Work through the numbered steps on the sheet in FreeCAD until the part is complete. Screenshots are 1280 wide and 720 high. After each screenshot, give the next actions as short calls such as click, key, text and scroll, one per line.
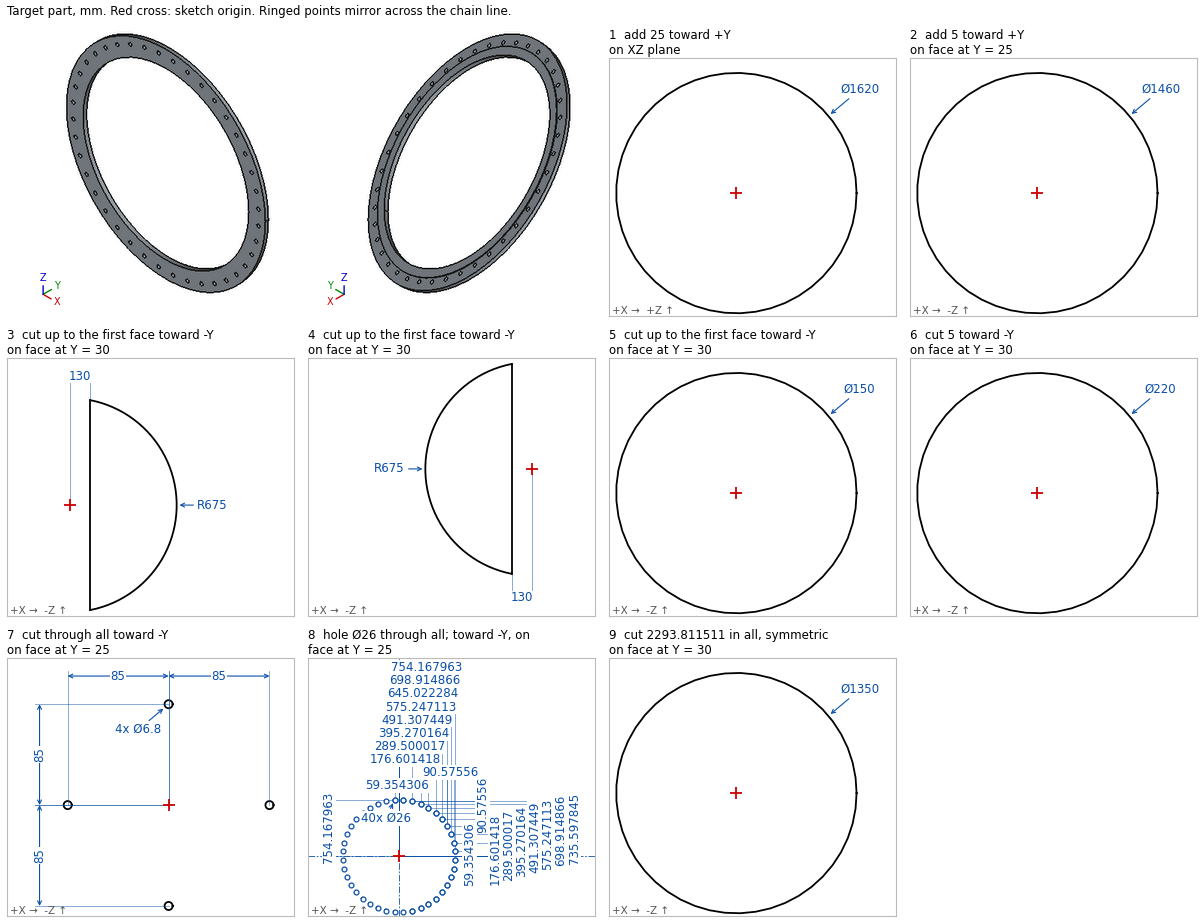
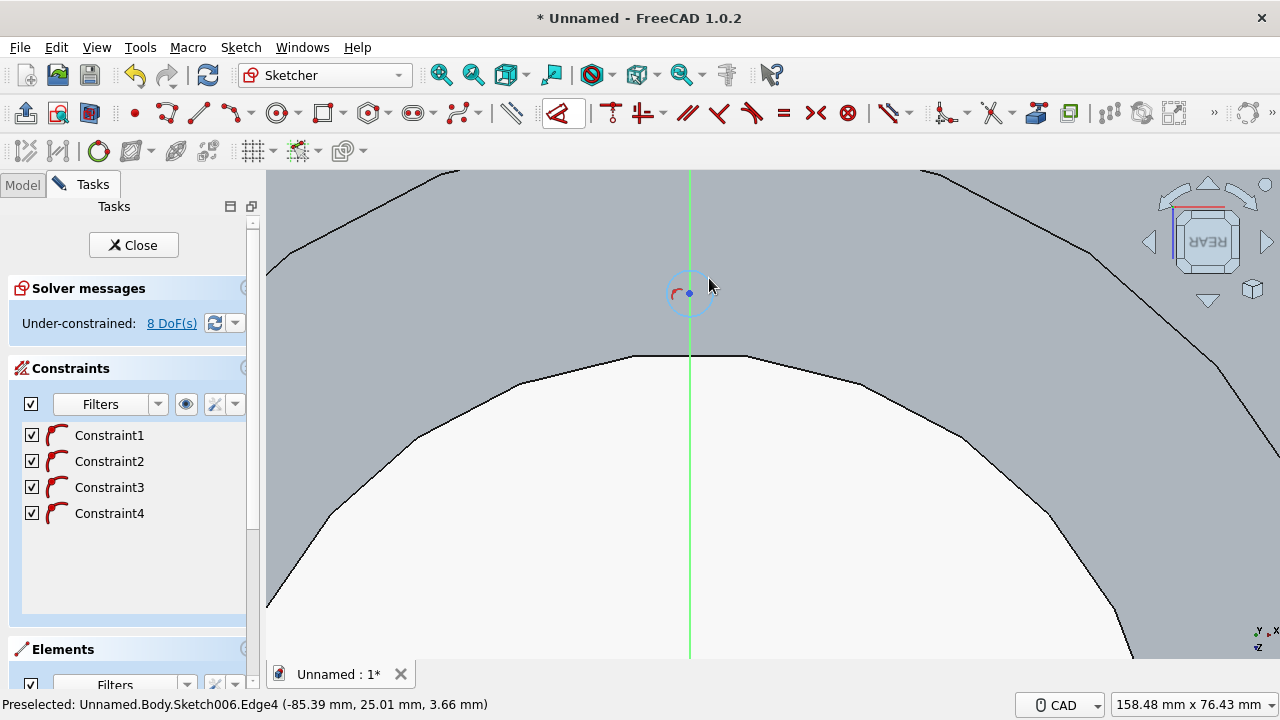
click(706, 277)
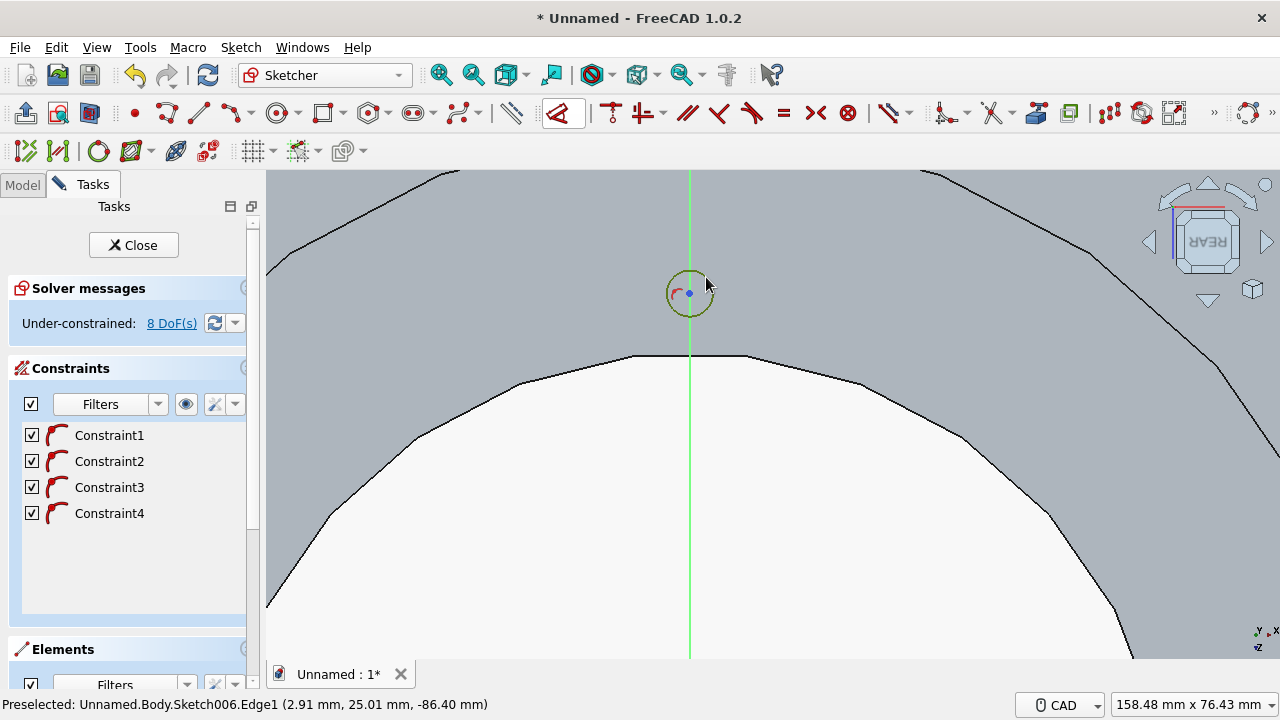
scroll(709, 278, down, 7)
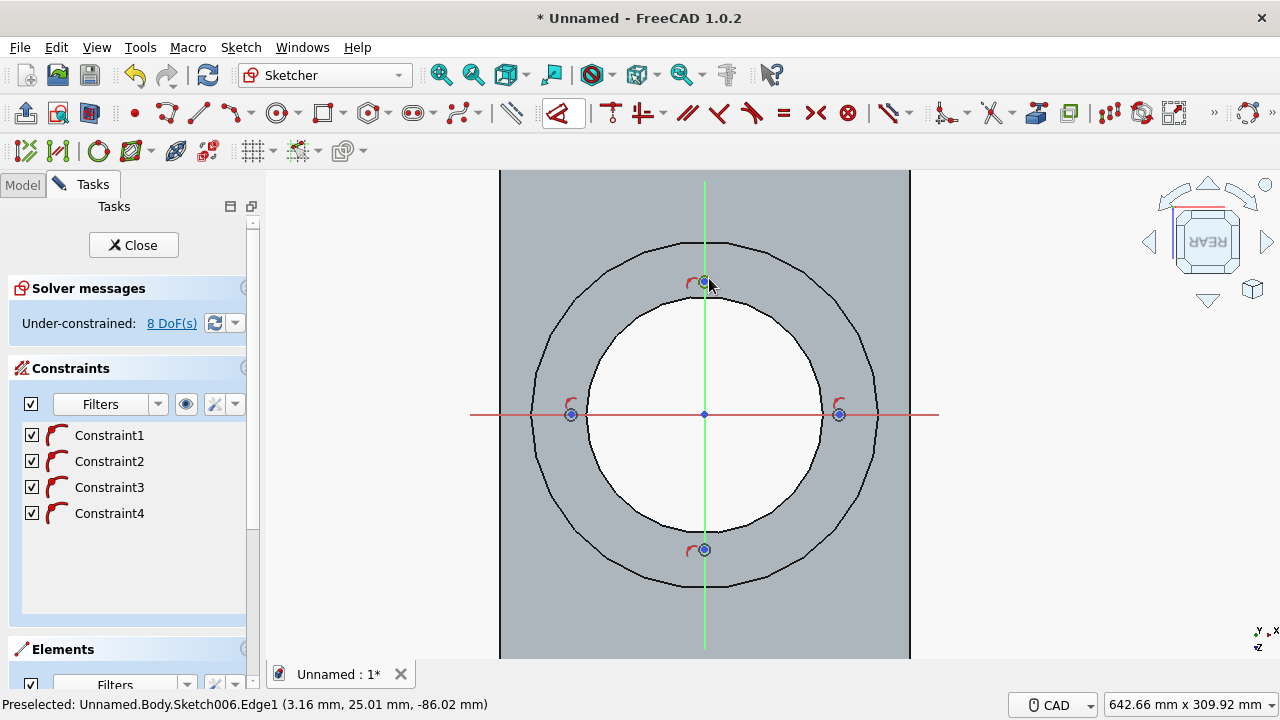
scroll(843, 411, up, 7)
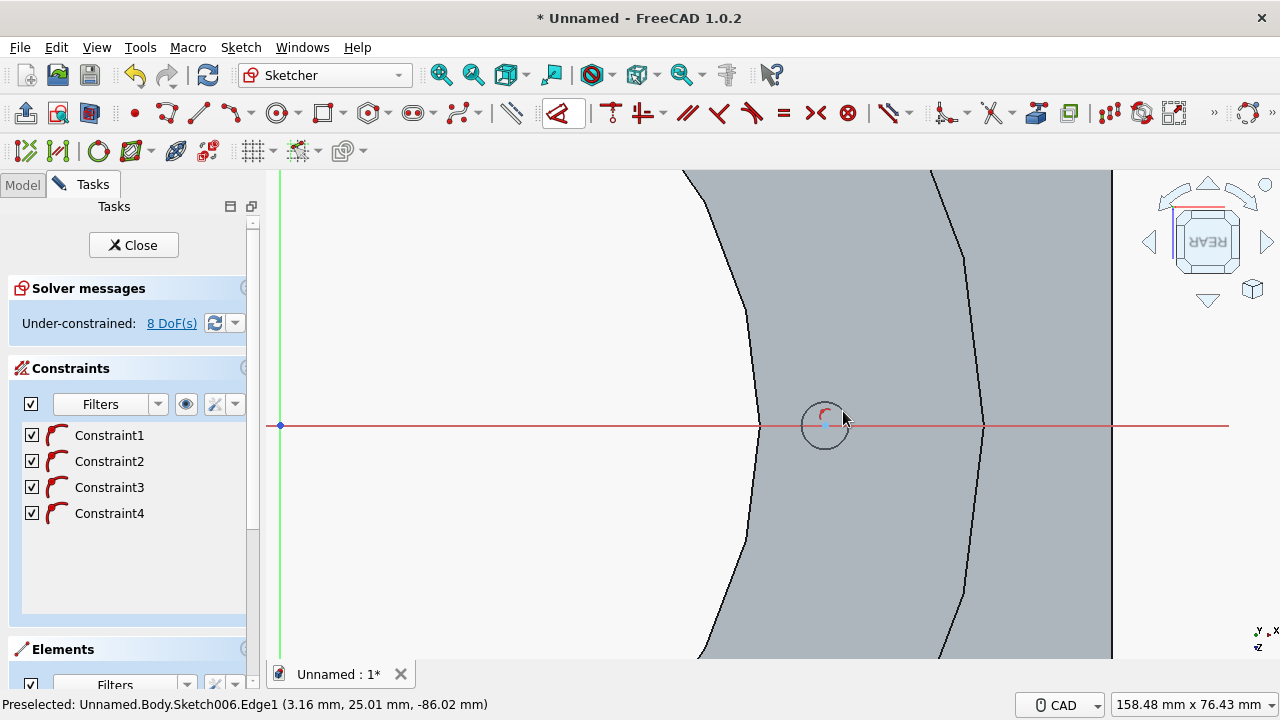
click(842, 409)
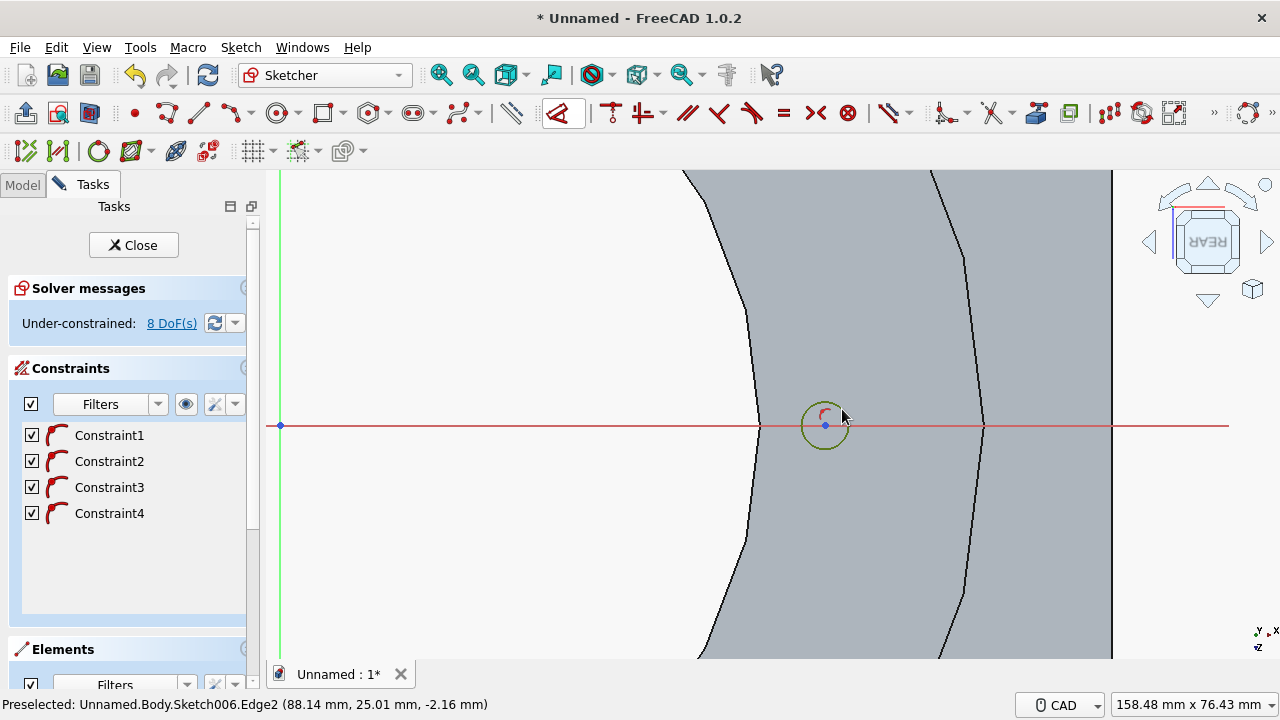
scroll(843, 411, down, 7)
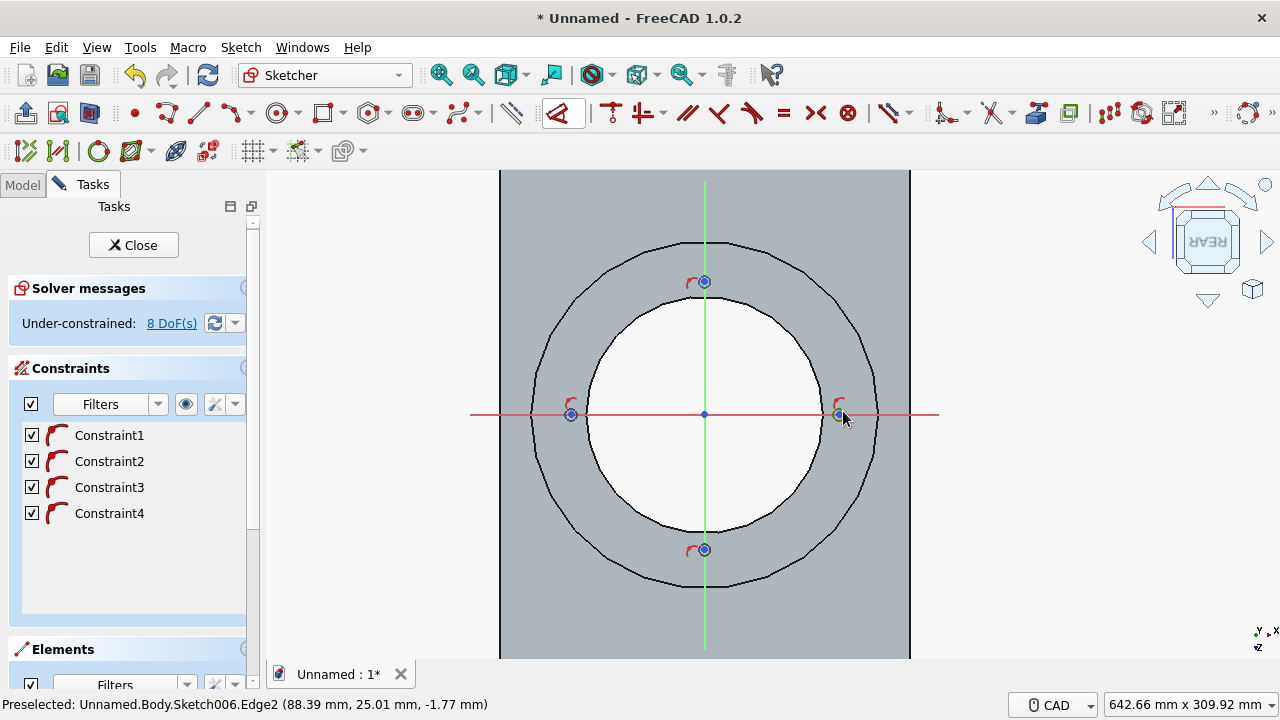
scroll(709, 546, up, 7)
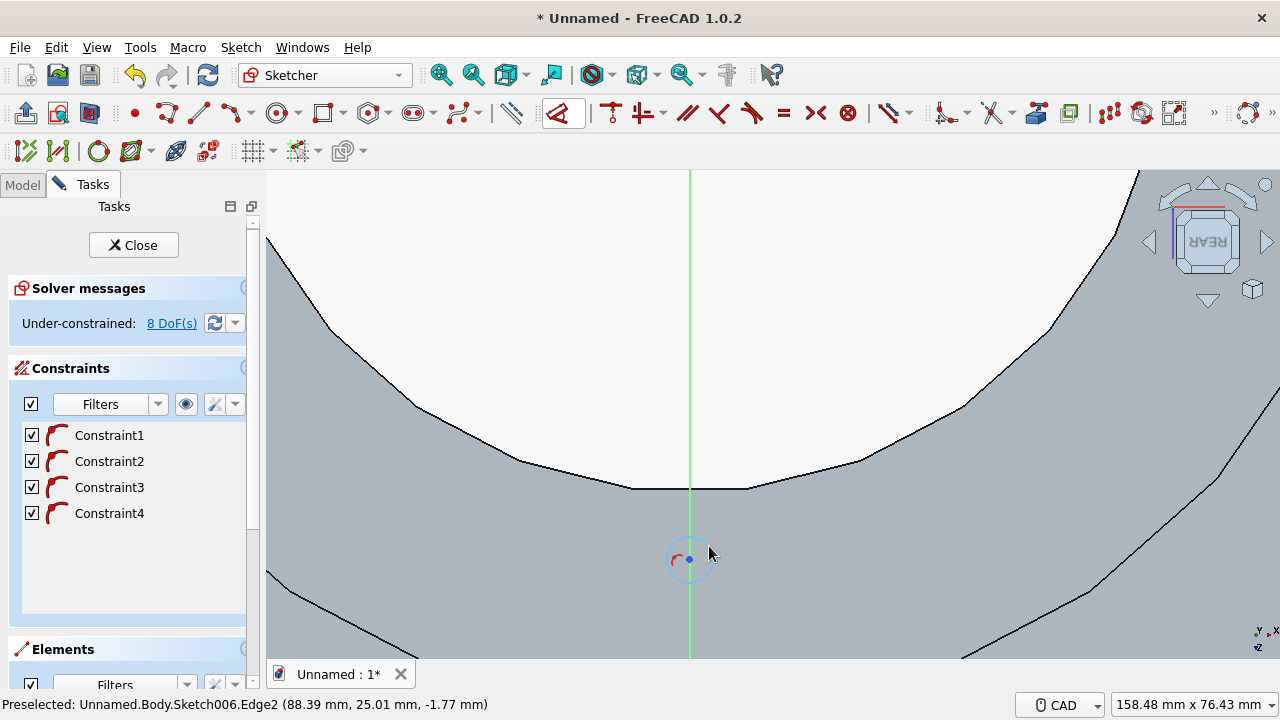
click(706, 544)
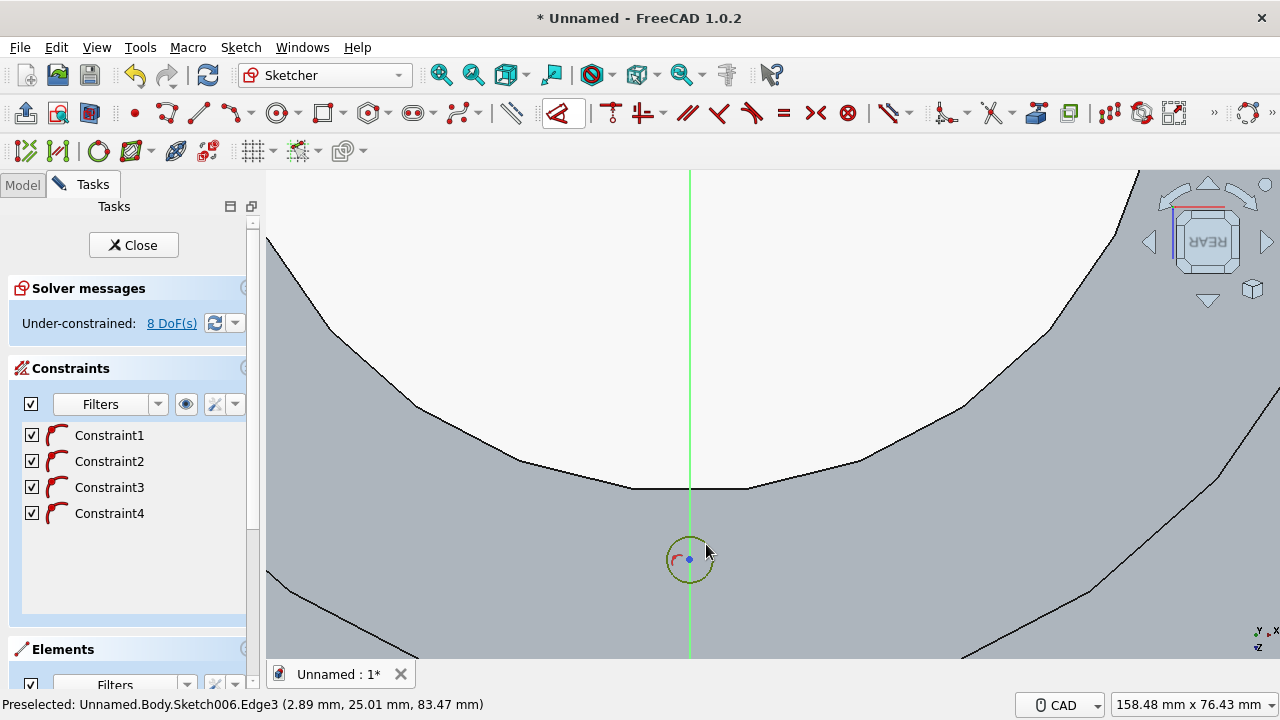
scroll(709, 546, down, 7)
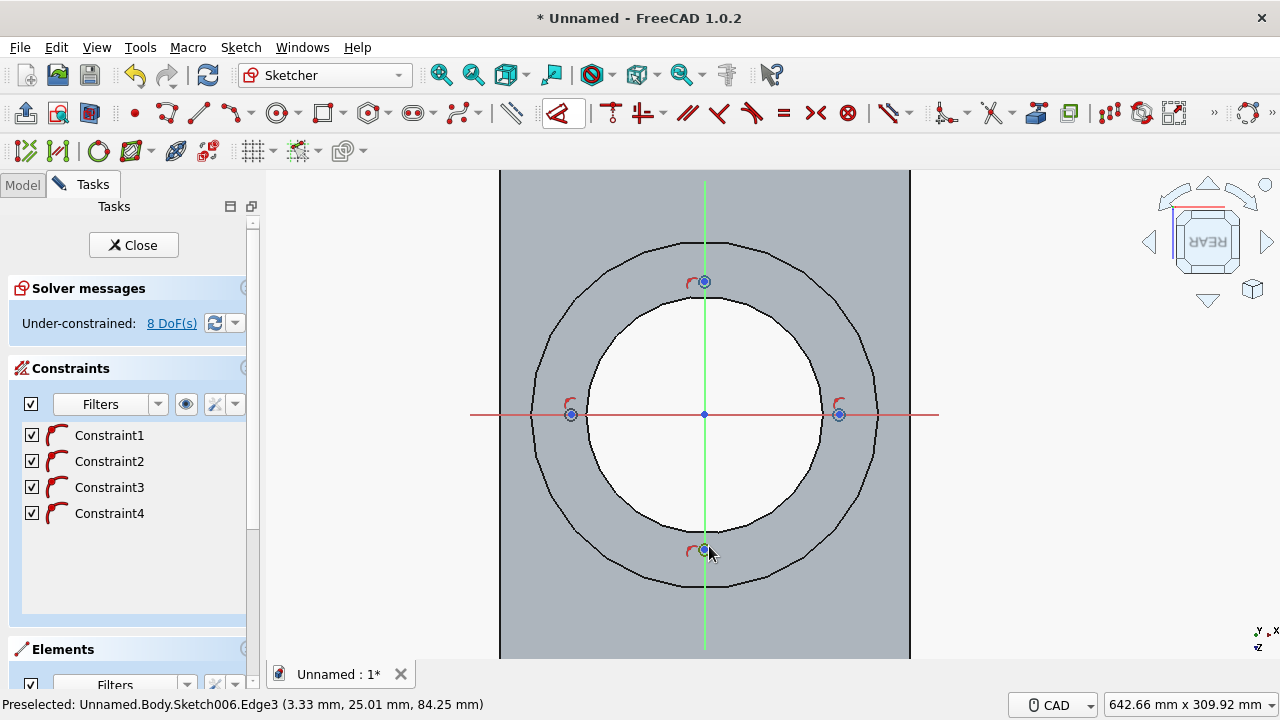
scroll(575, 411, up, 6)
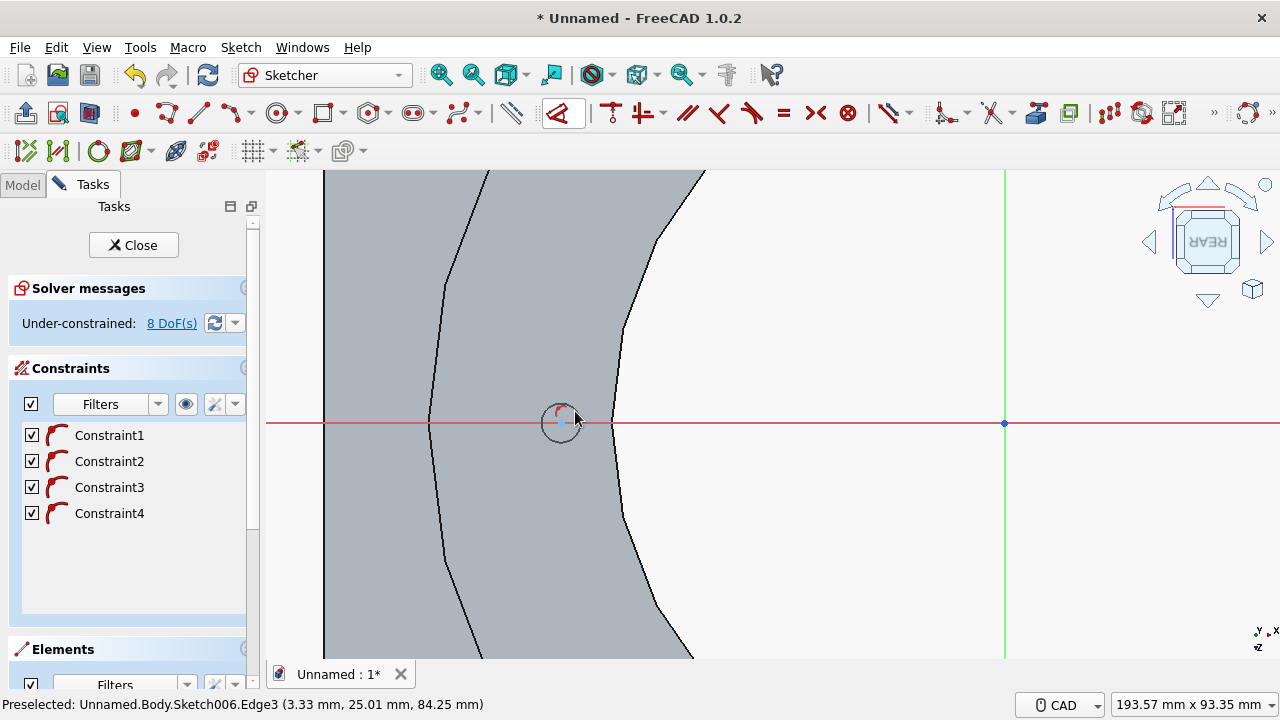
click(575, 409)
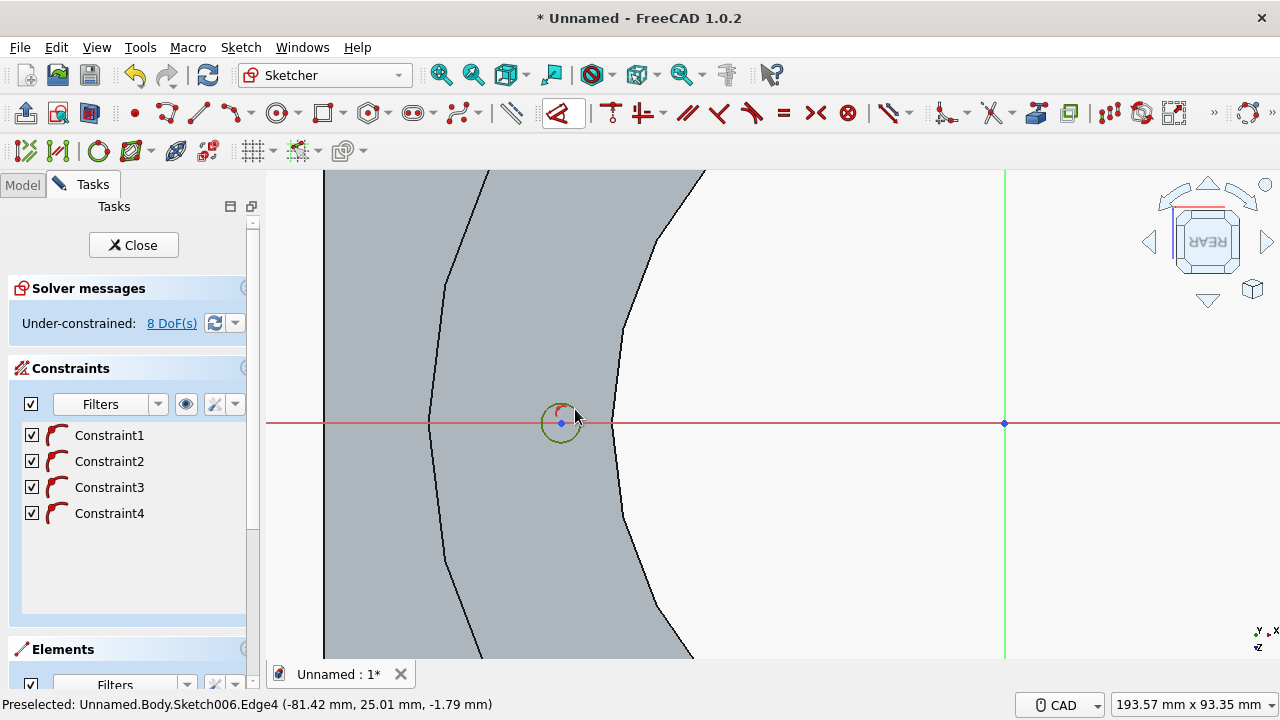
click(784, 114)